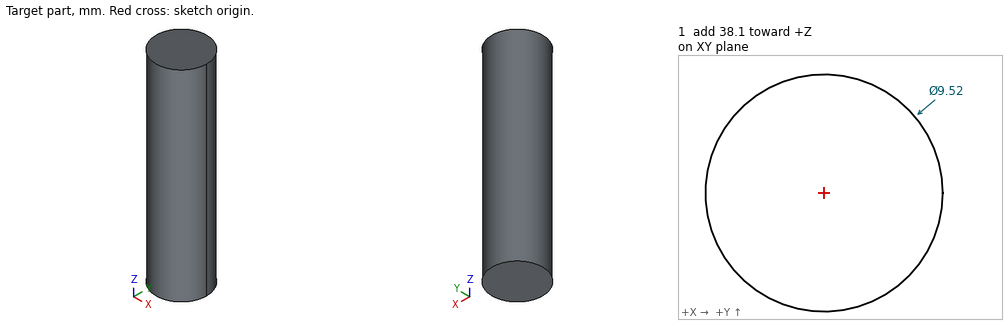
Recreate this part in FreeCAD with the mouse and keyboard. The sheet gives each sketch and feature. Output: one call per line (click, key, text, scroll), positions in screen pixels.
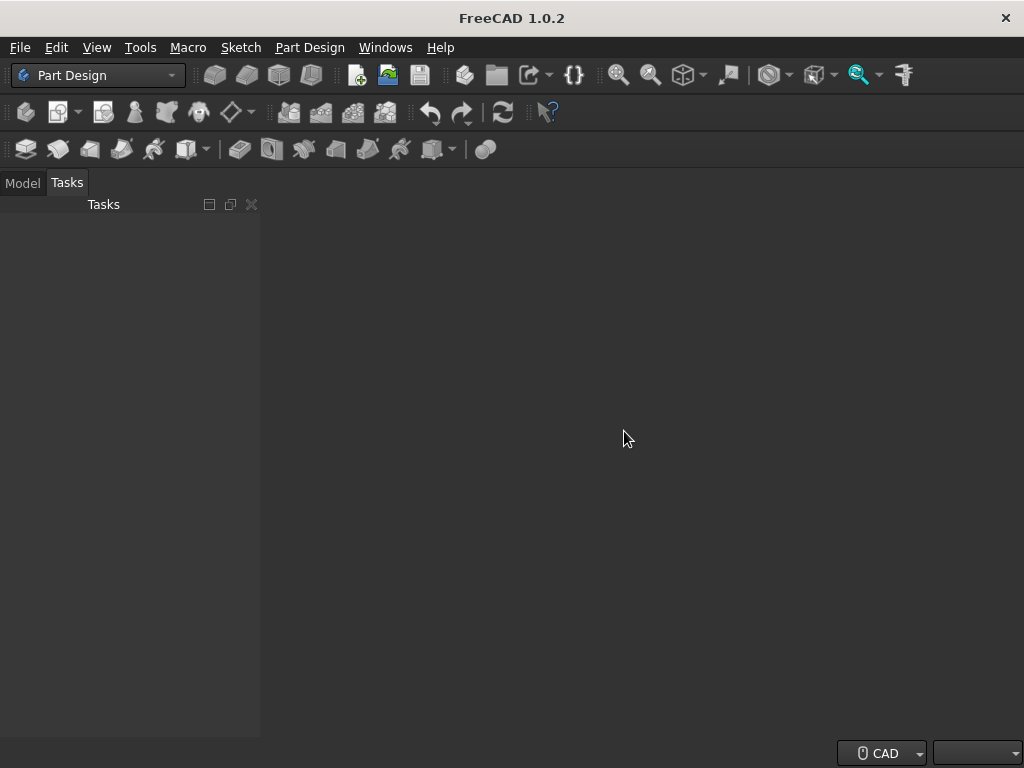
click(356, 76)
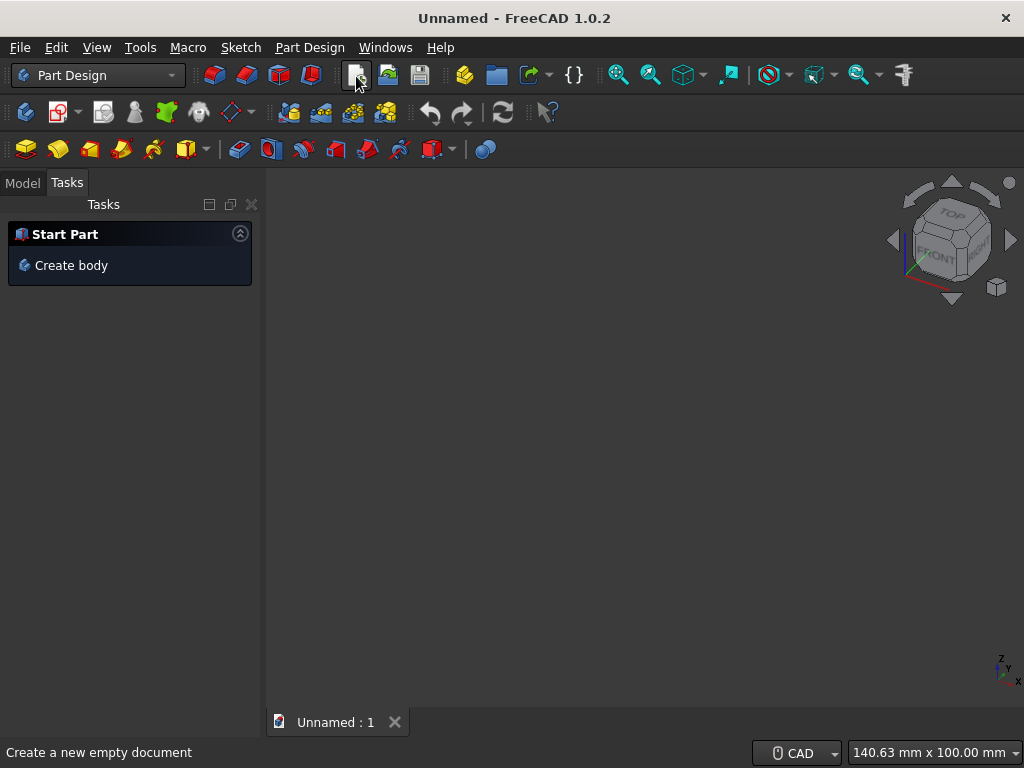
click(58, 112)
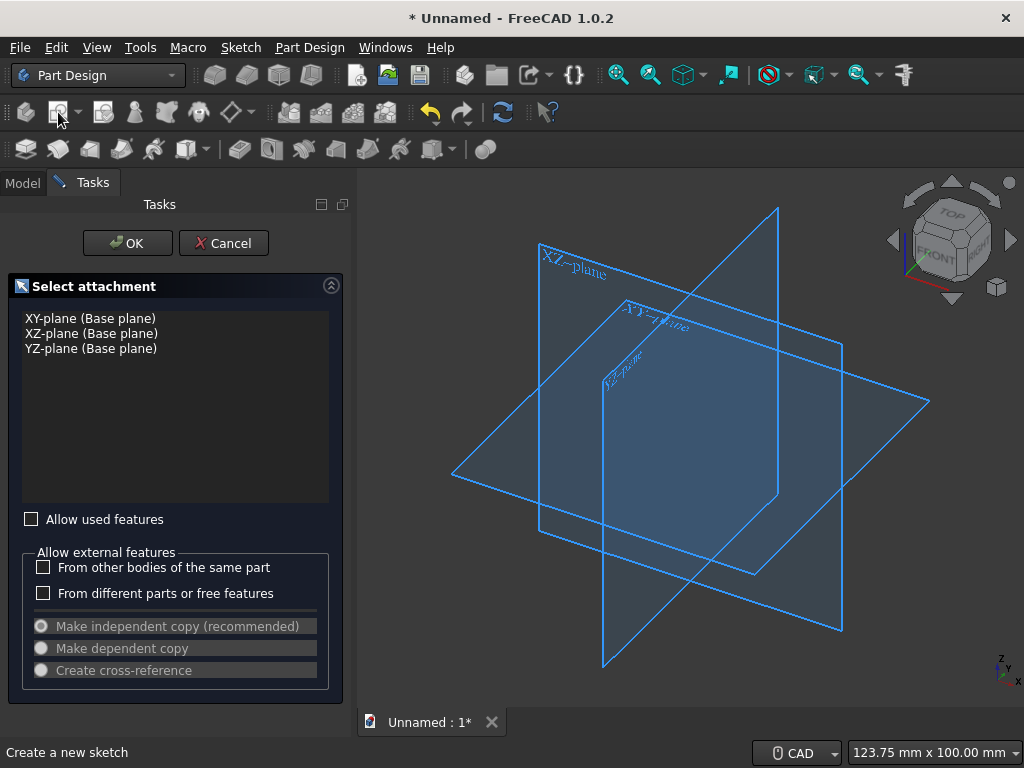
click(82, 318)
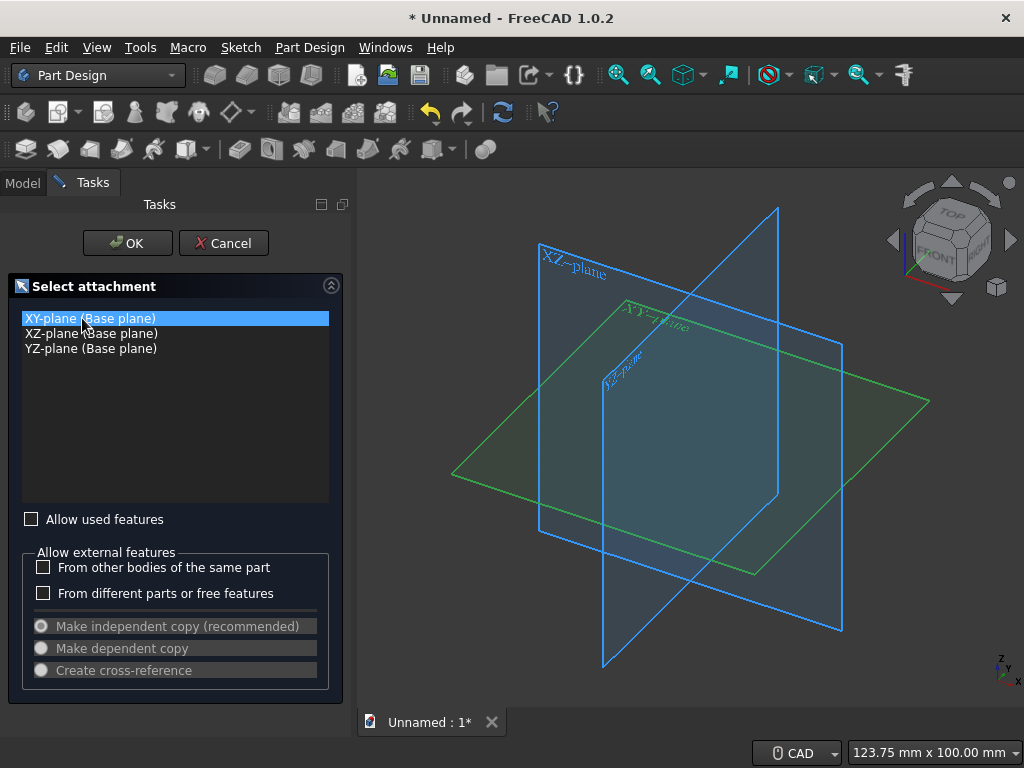
click(128, 243)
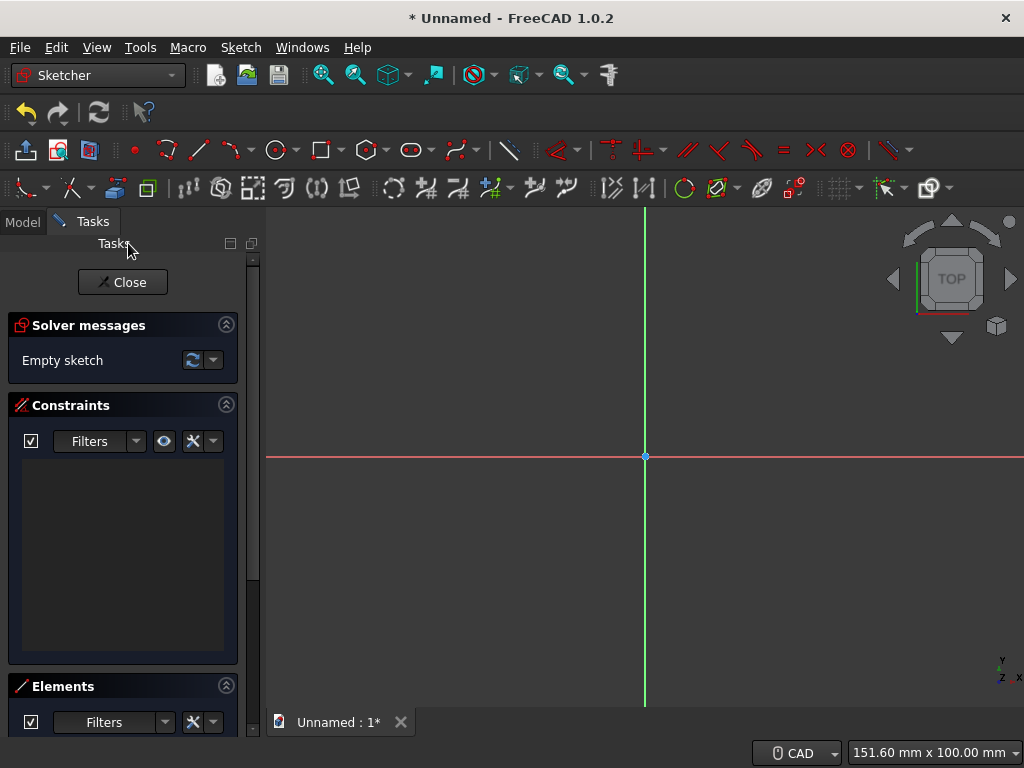
scroll(659, 457, up, 9)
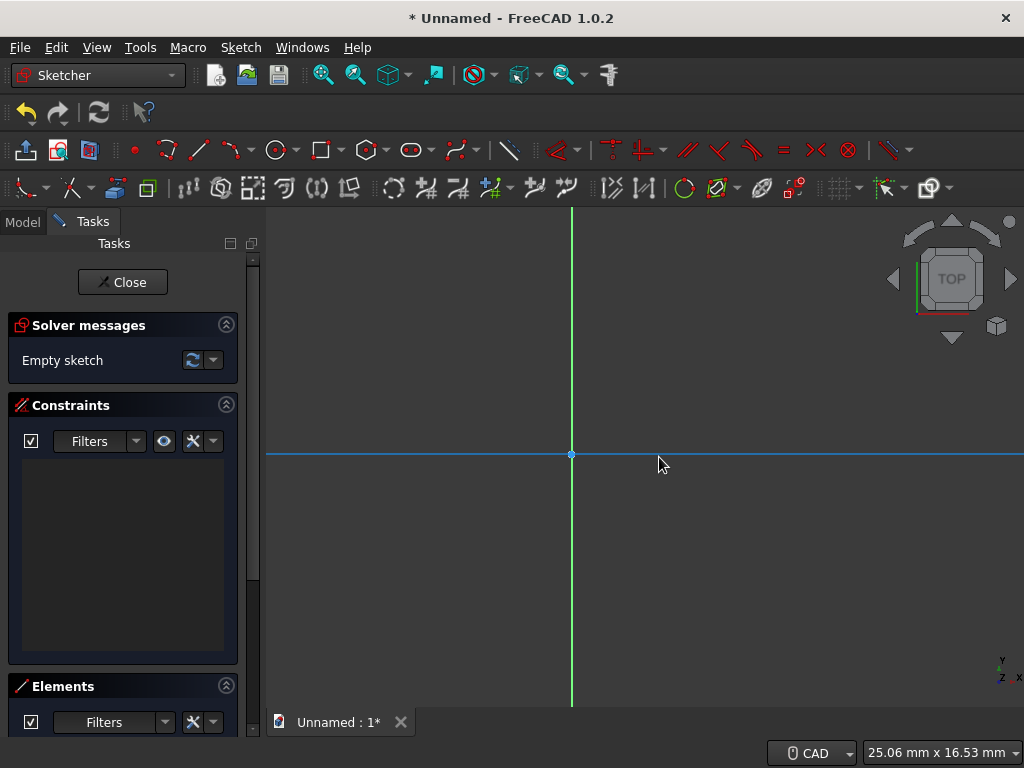
key(g)
key(c)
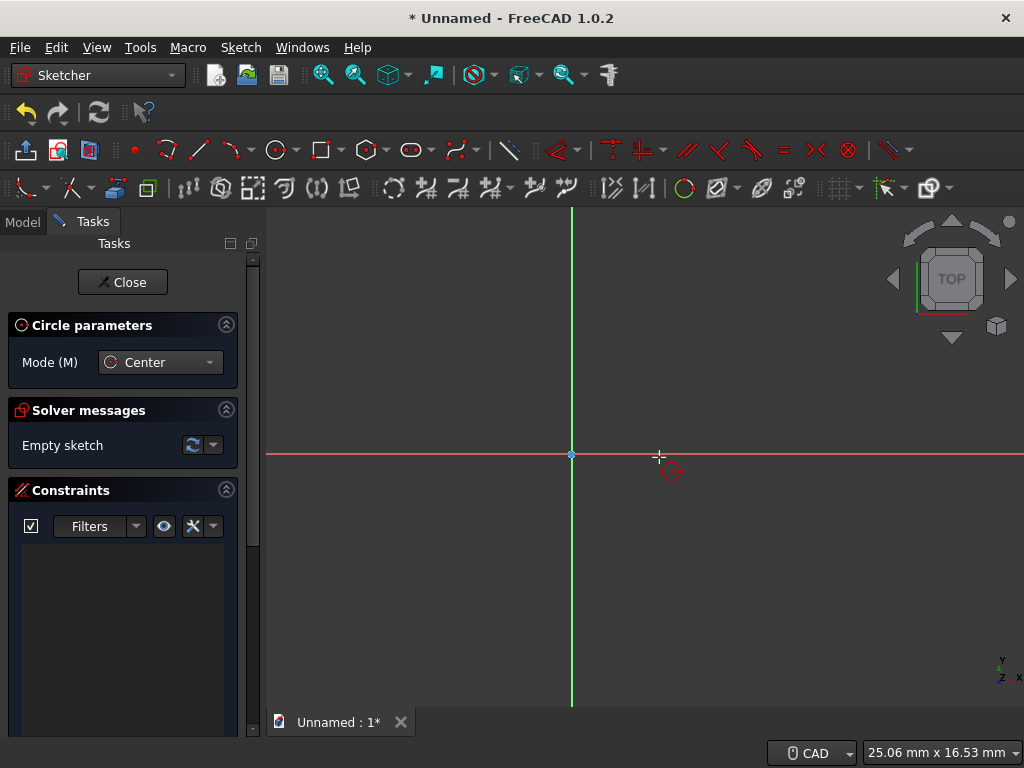
click(572, 454)
move(673, 353)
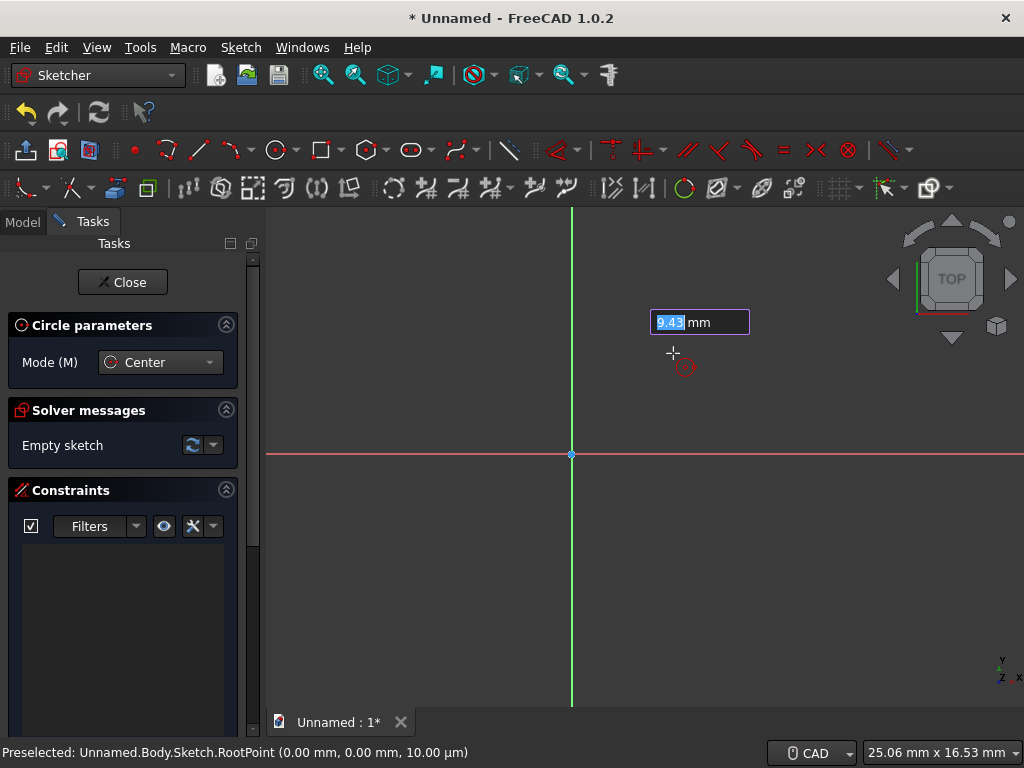
text(9.52)
key(Return)
key(Escape)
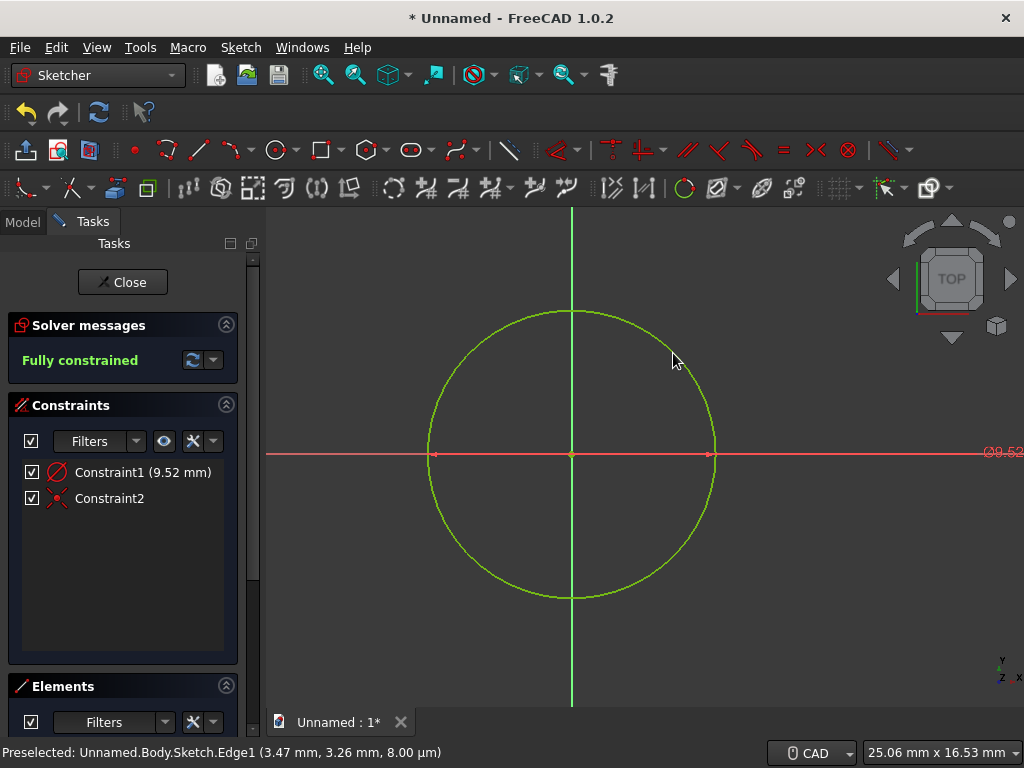
click(123, 282)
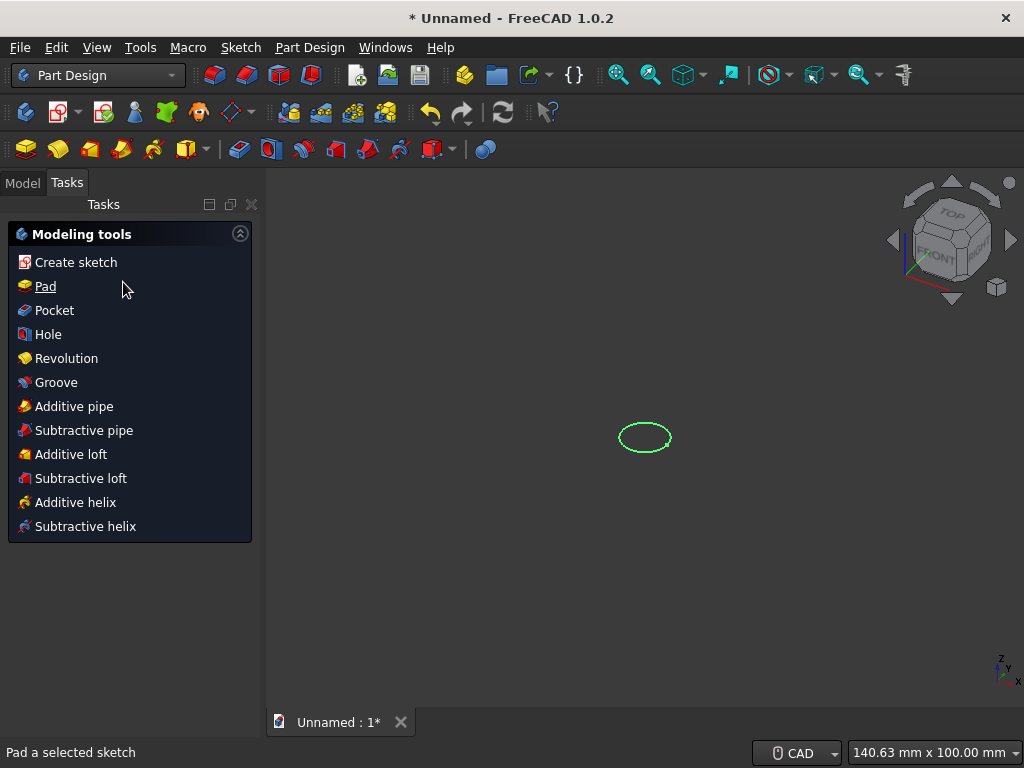
click(26, 150)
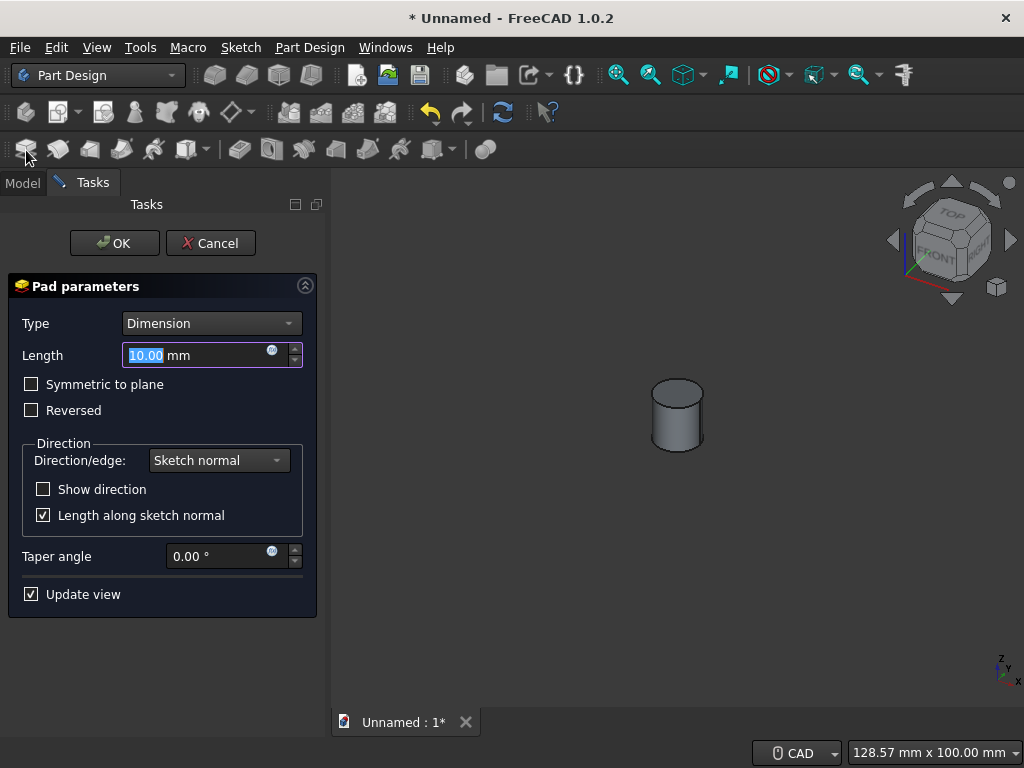
text(38.1)
key(Tab)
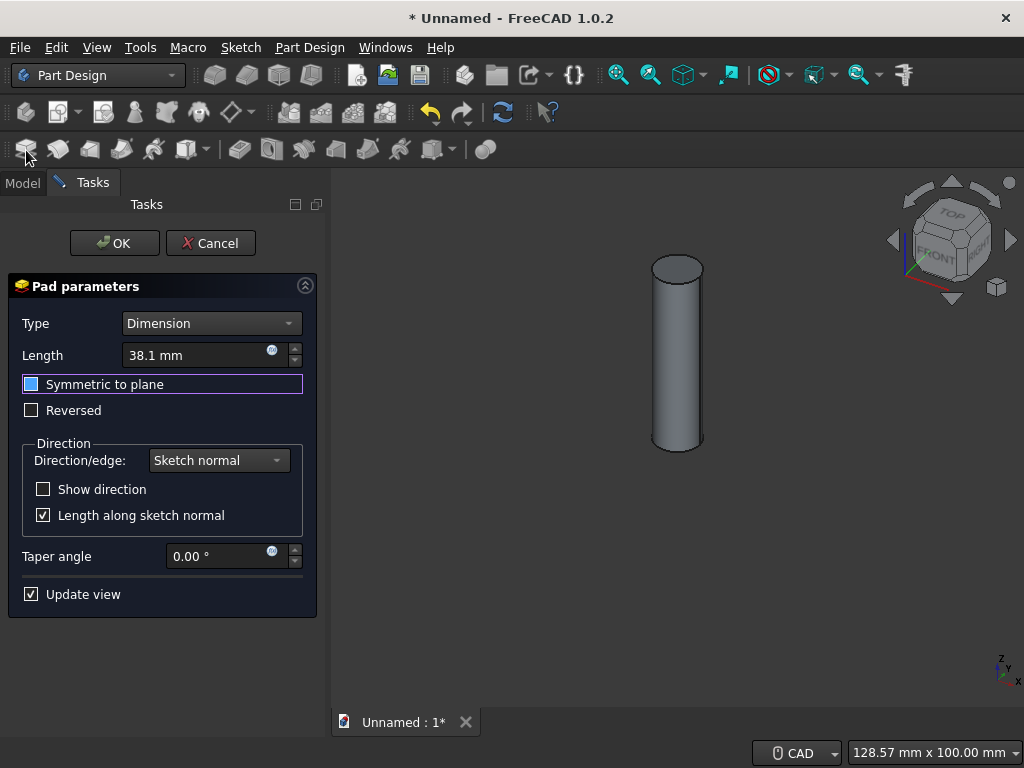
click(115, 243)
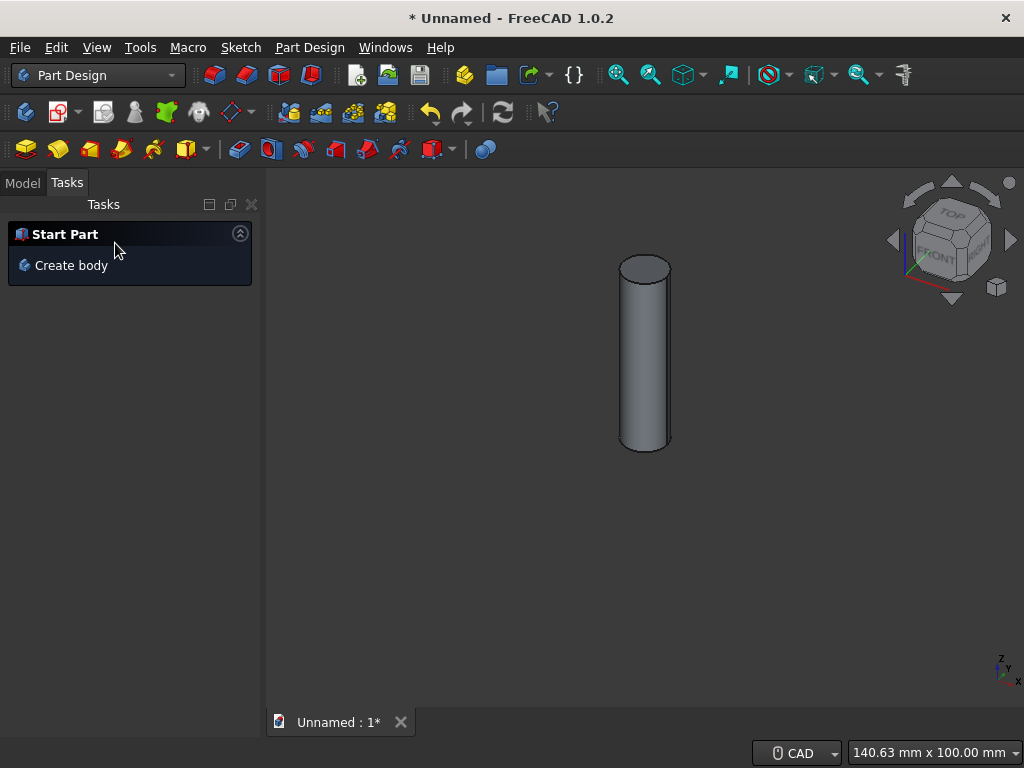
key(0)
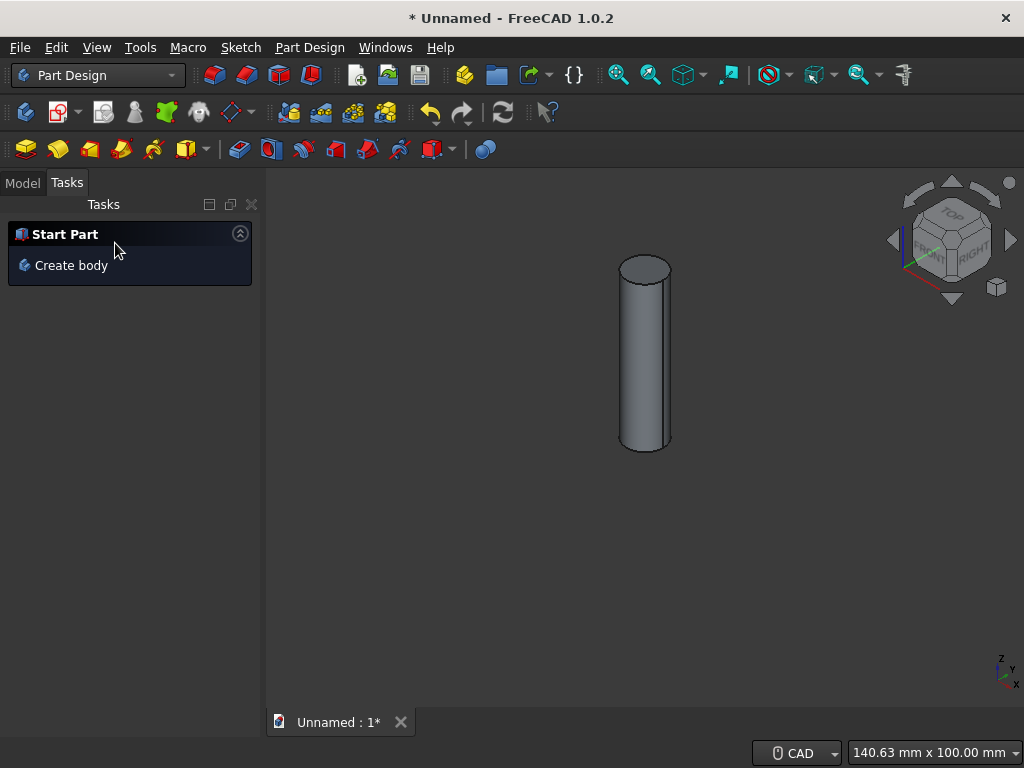
key(v)
key(f)